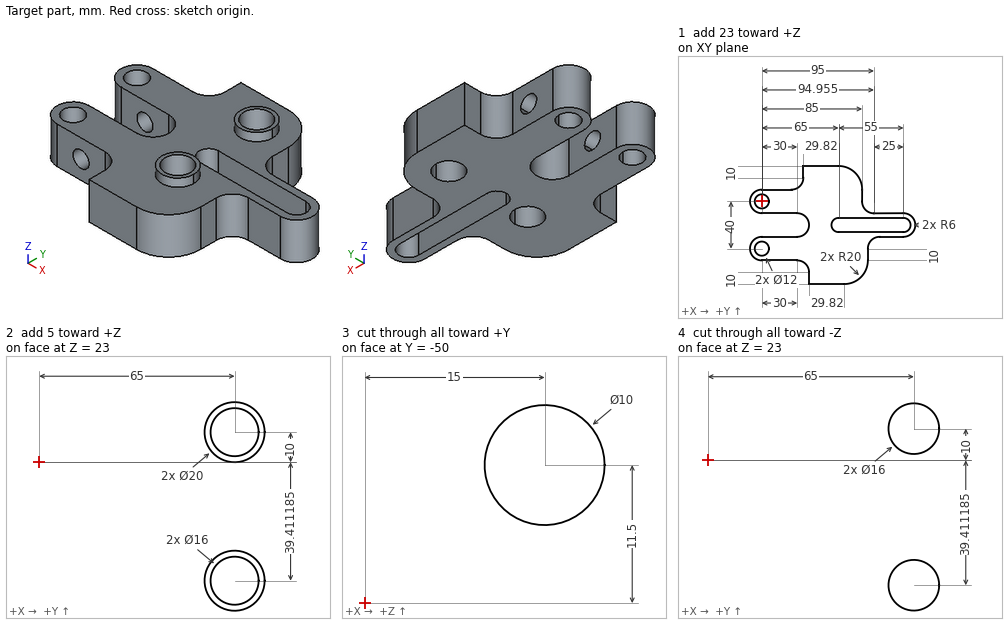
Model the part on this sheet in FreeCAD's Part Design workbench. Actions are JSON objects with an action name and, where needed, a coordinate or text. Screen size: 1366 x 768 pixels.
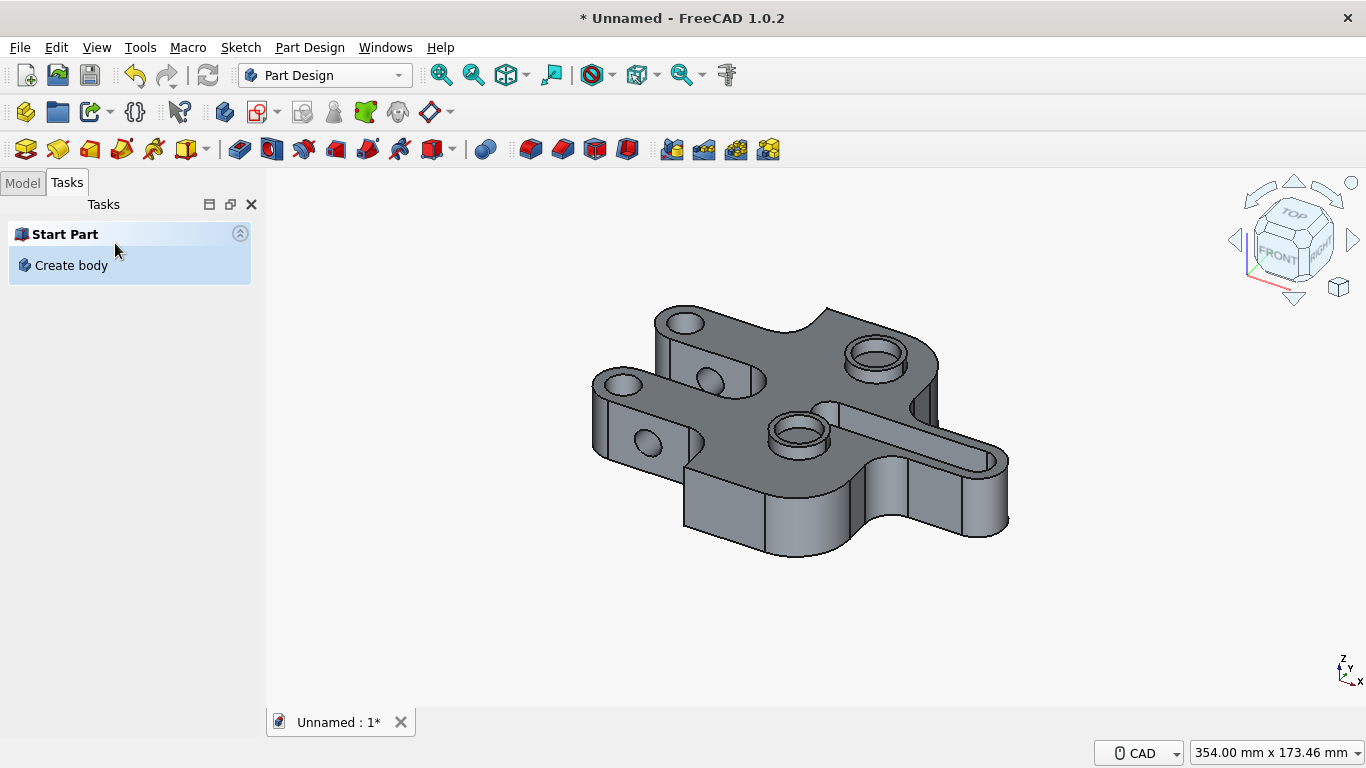
{"action": "left_click", "coordinate": [807, 345]}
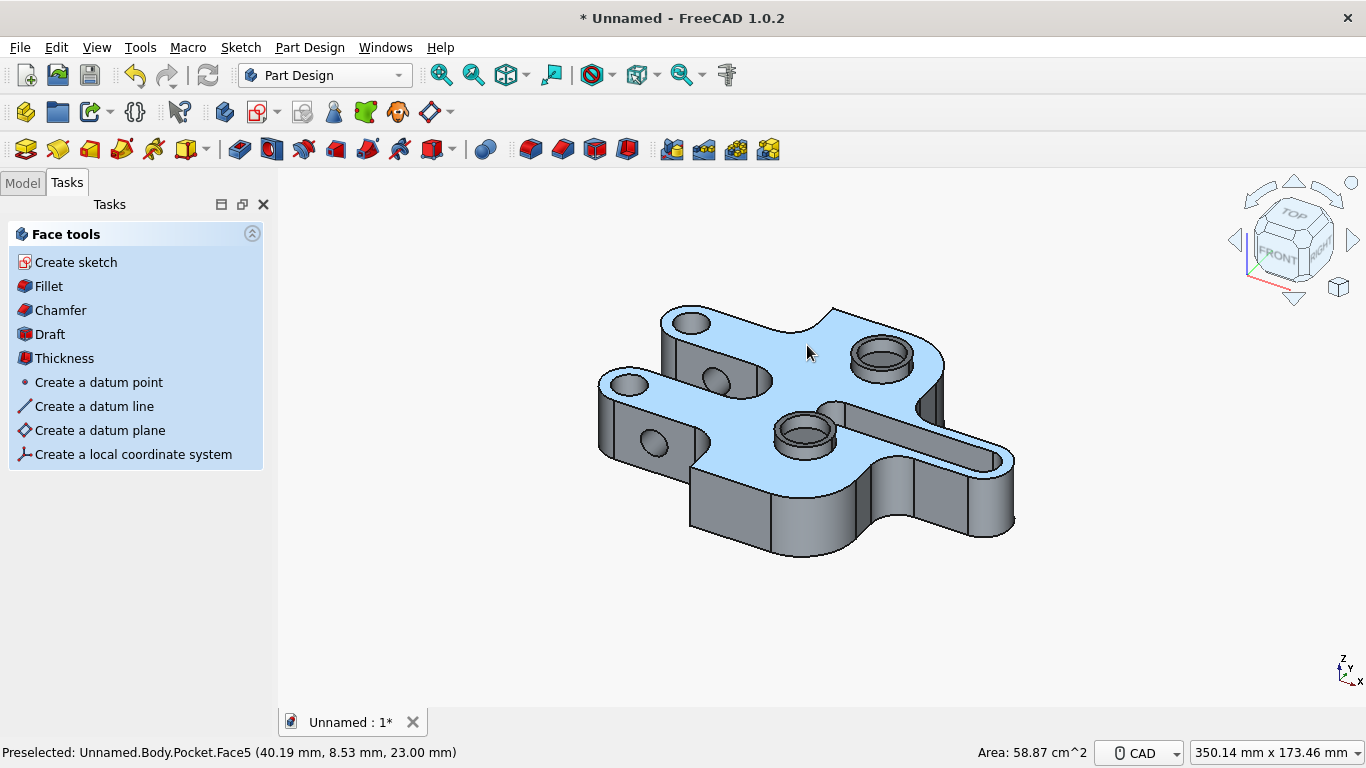
{"action": "left_click", "coordinate": [258, 112]}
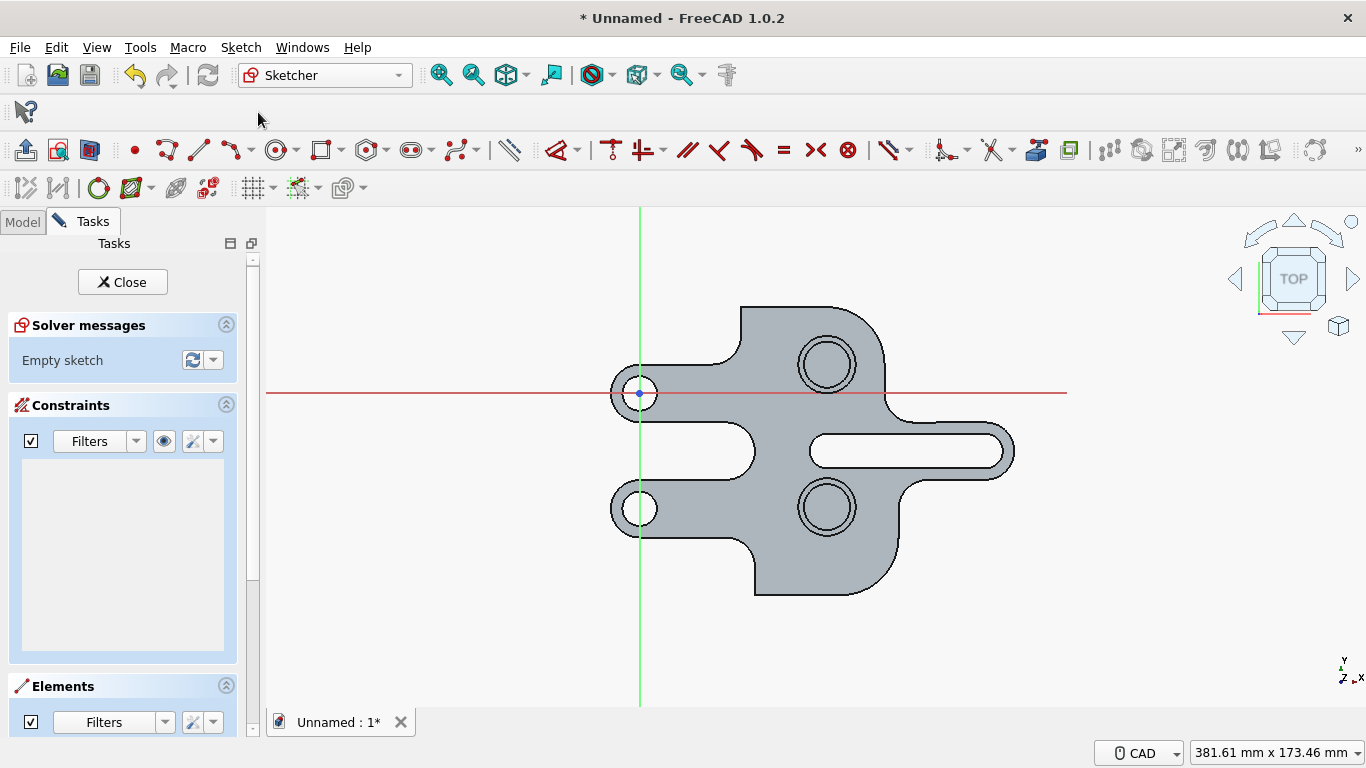
{"action": "left_click", "coordinate": [90, 150]}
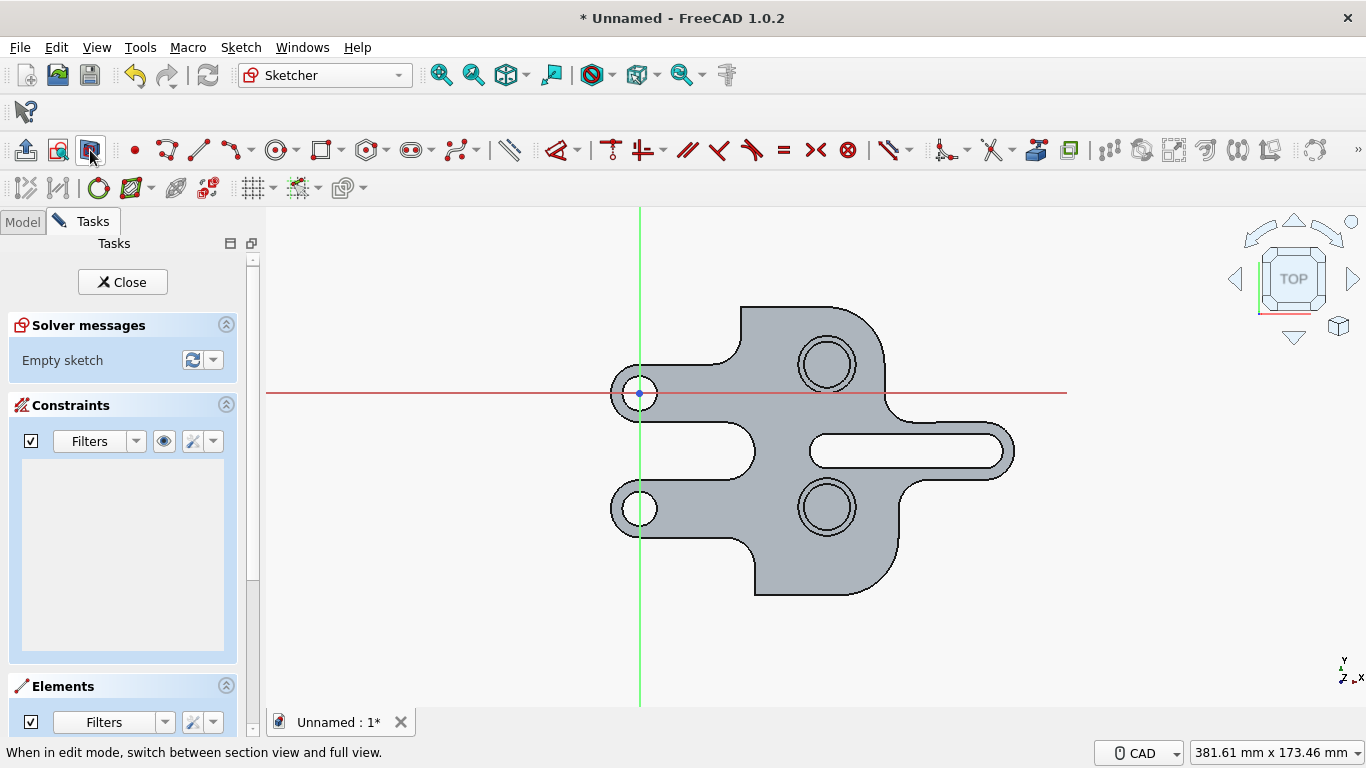
{"action": "scroll", "coordinate": [742, 410], "scroll_direction": "up", "scroll_amount": 3}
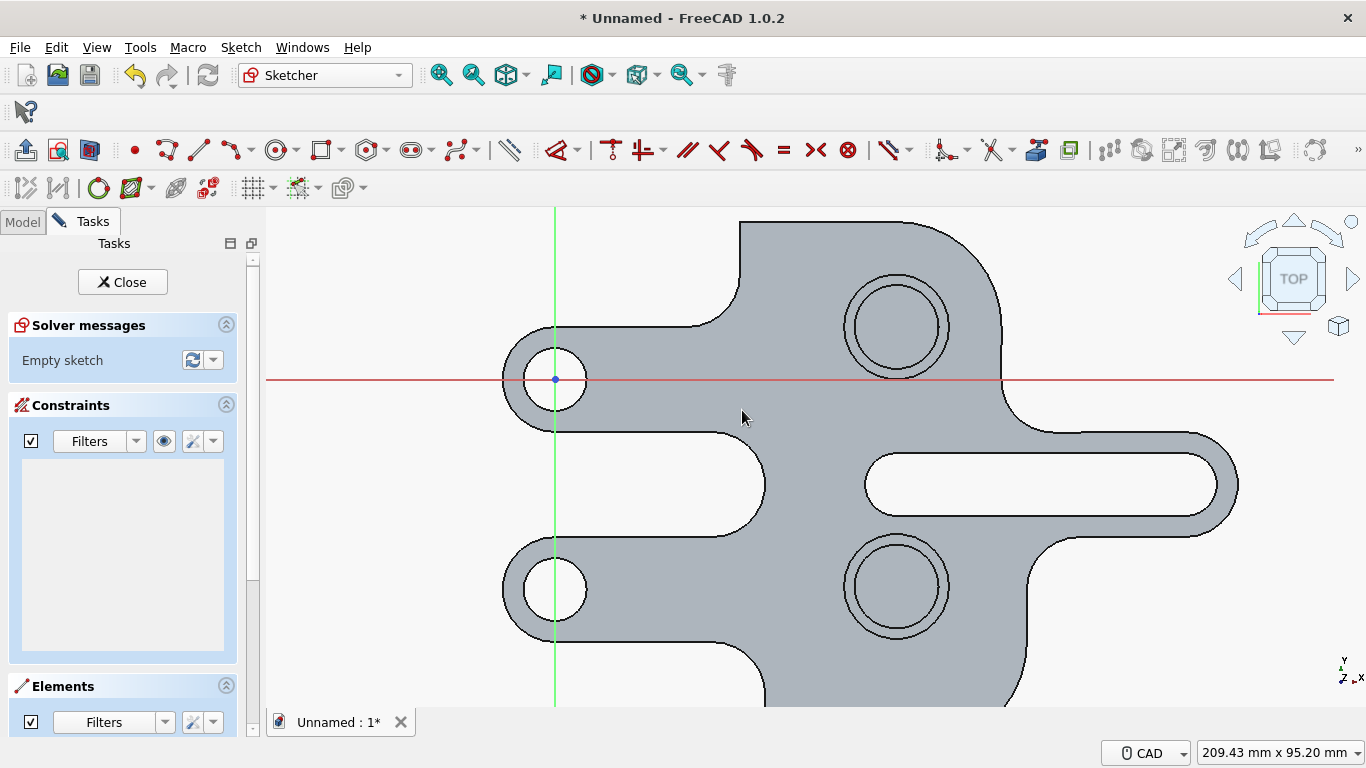
{"action": "key", "text": "g c"}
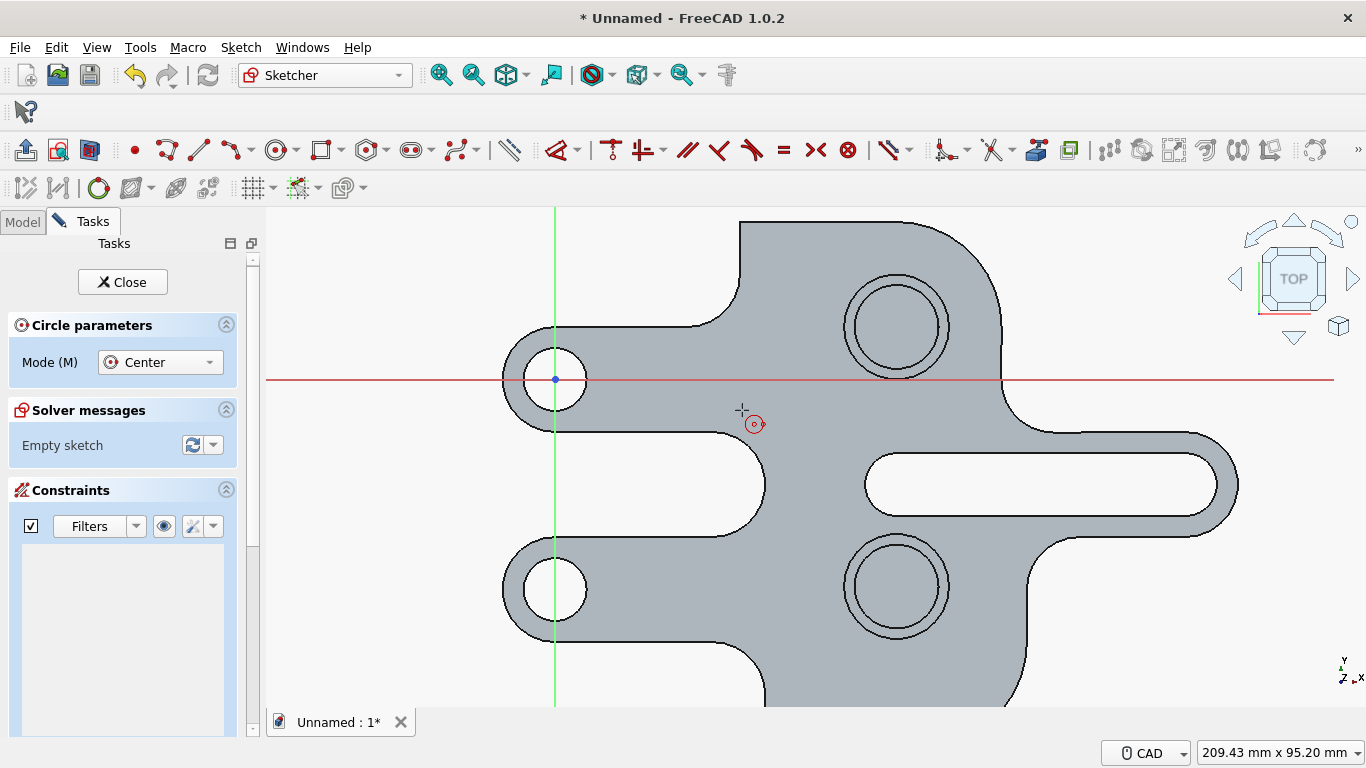
{"action": "left_click", "coordinate": [897, 327]}
{"action": "mouse_move", "coordinate": [926, 297]}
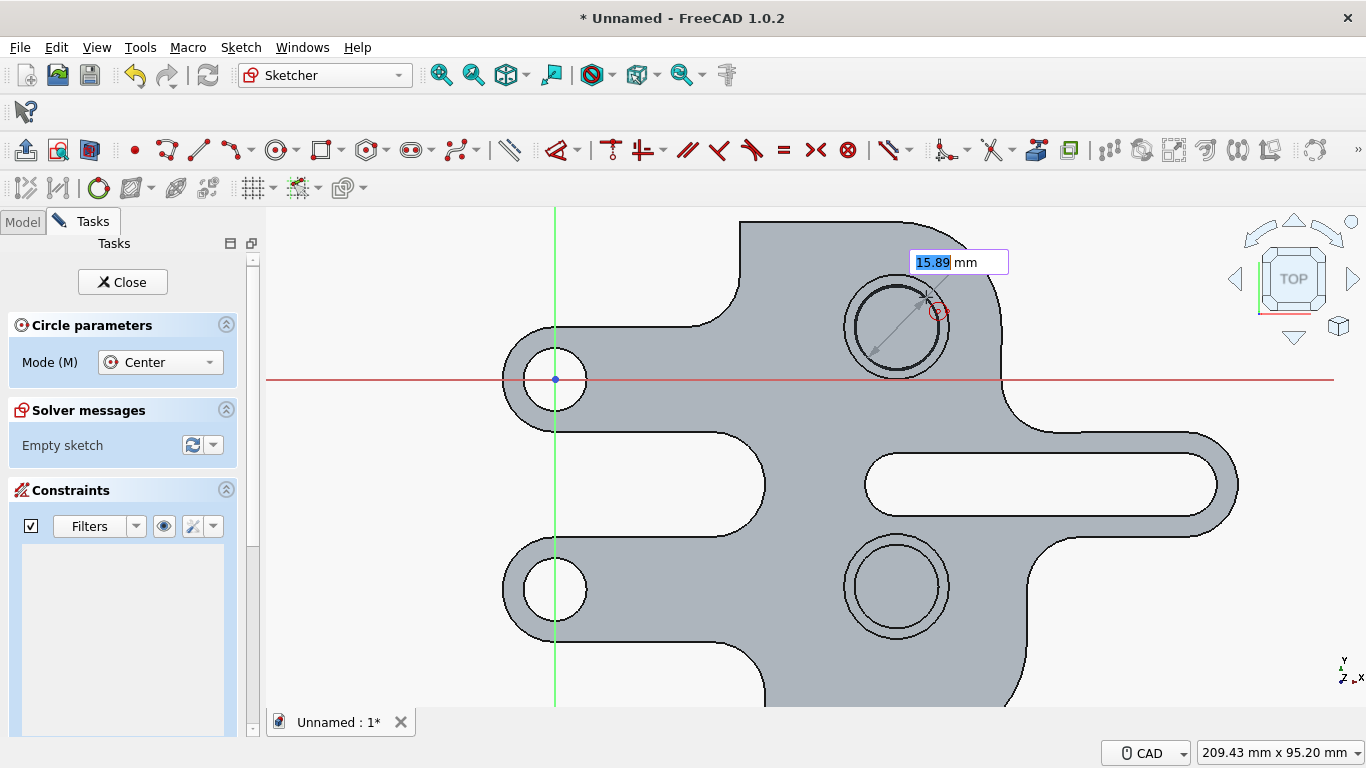
{"action": "type", "text": "16"}
{"action": "key", "text": "Return"}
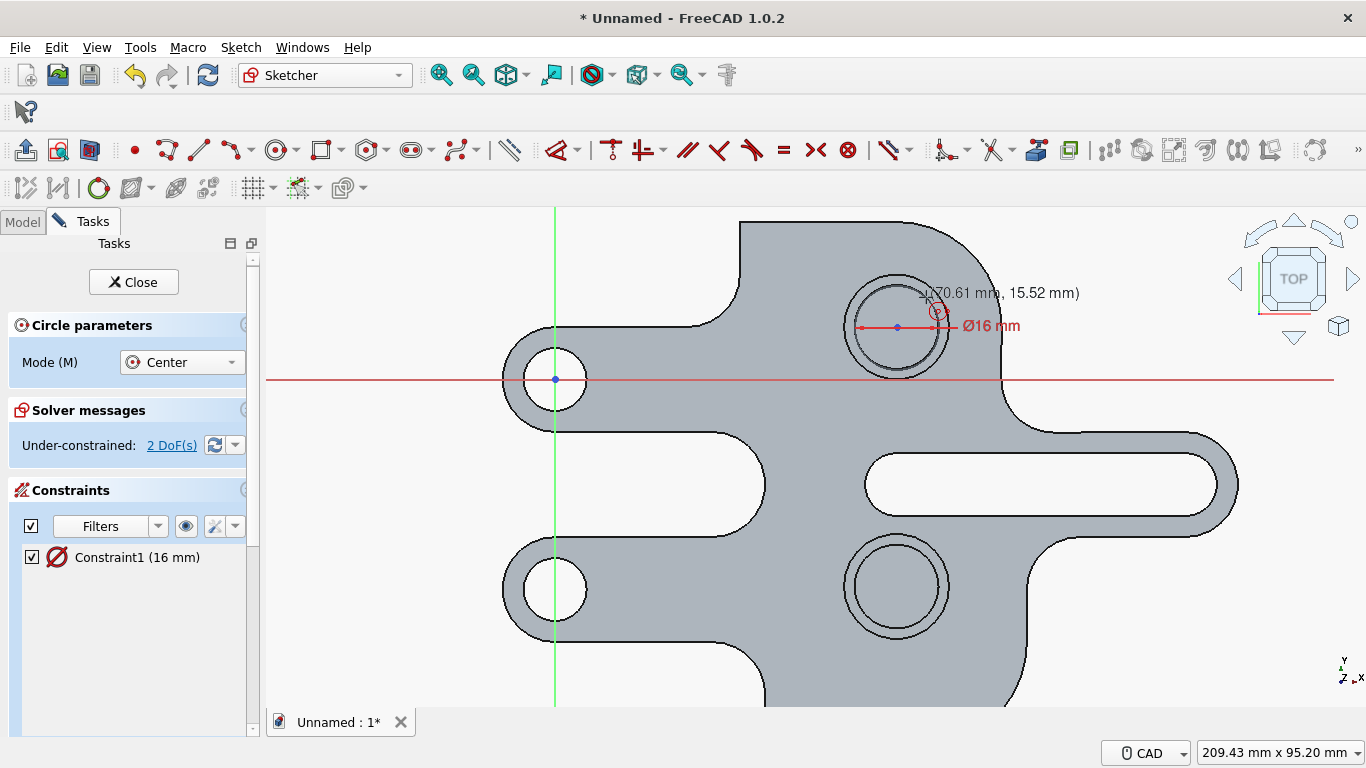
{"action": "left_click", "coordinate": [897, 587]}
{"action": "mouse_move", "coordinate": [926, 557]}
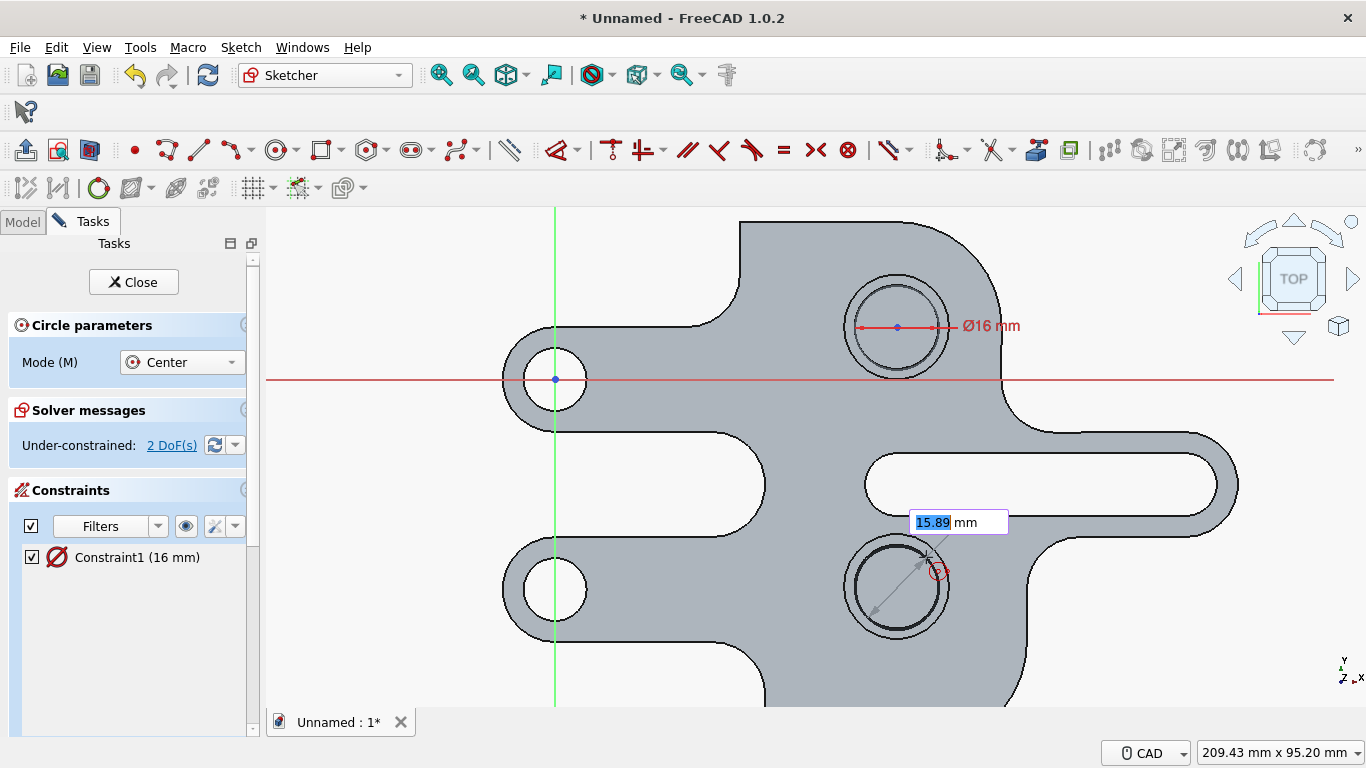
{"action": "type", "text": "16"}
{"action": "key", "text": "Return"}
{"action": "key", "text": "Escape"}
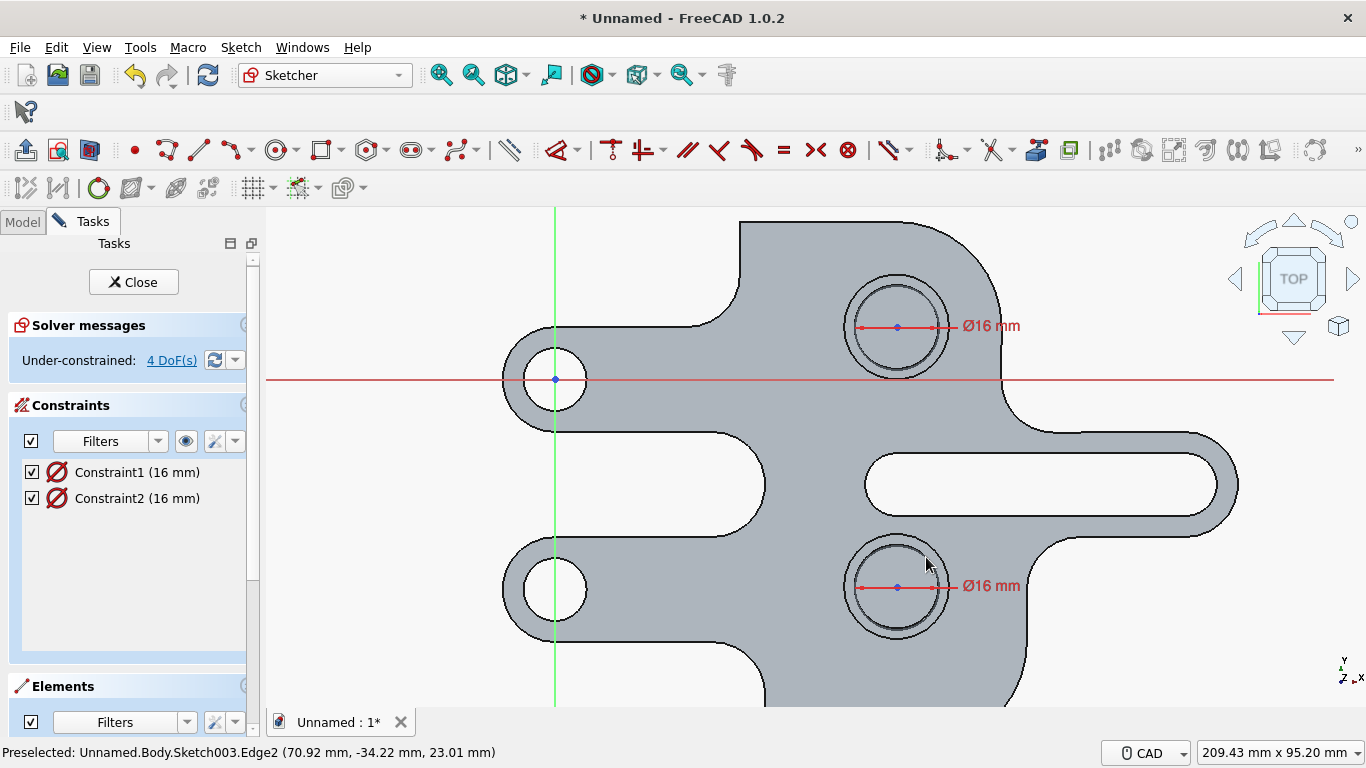
{"action": "left_click", "coordinate": [897, 328]}